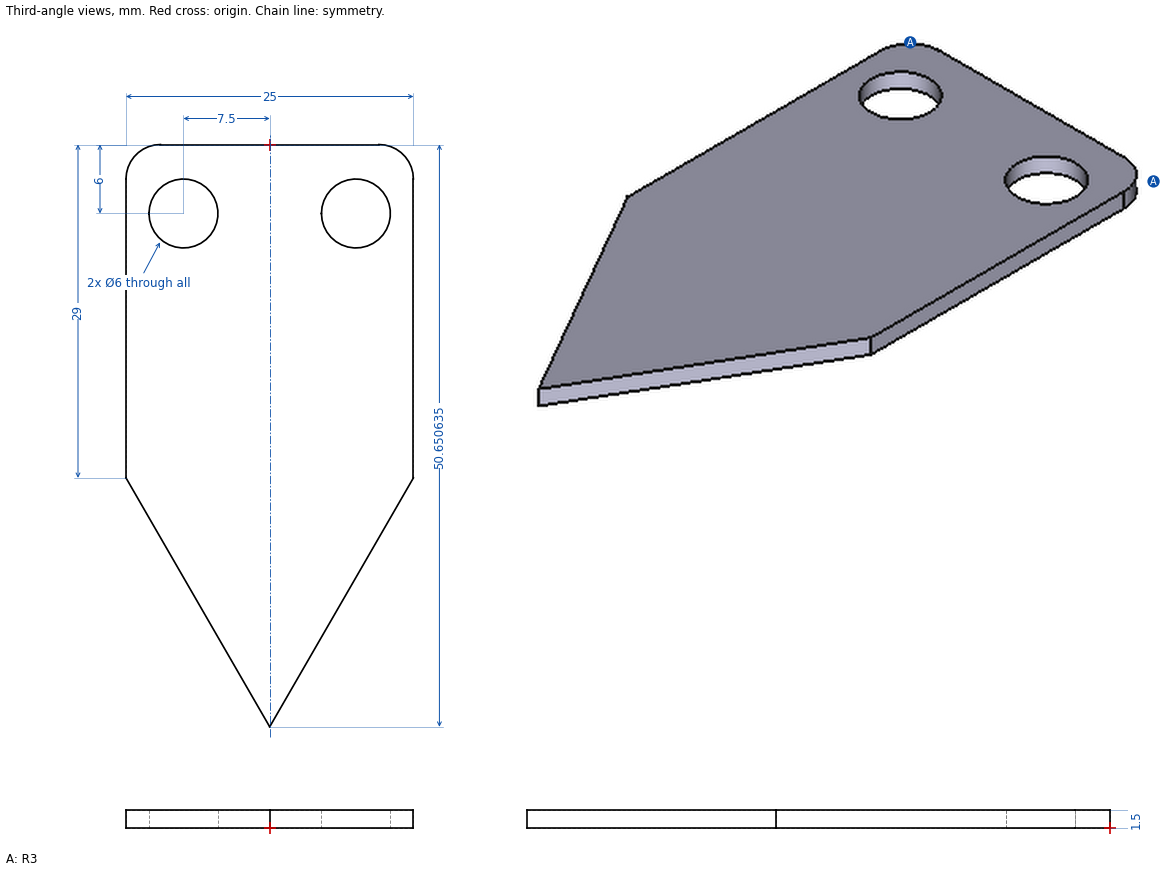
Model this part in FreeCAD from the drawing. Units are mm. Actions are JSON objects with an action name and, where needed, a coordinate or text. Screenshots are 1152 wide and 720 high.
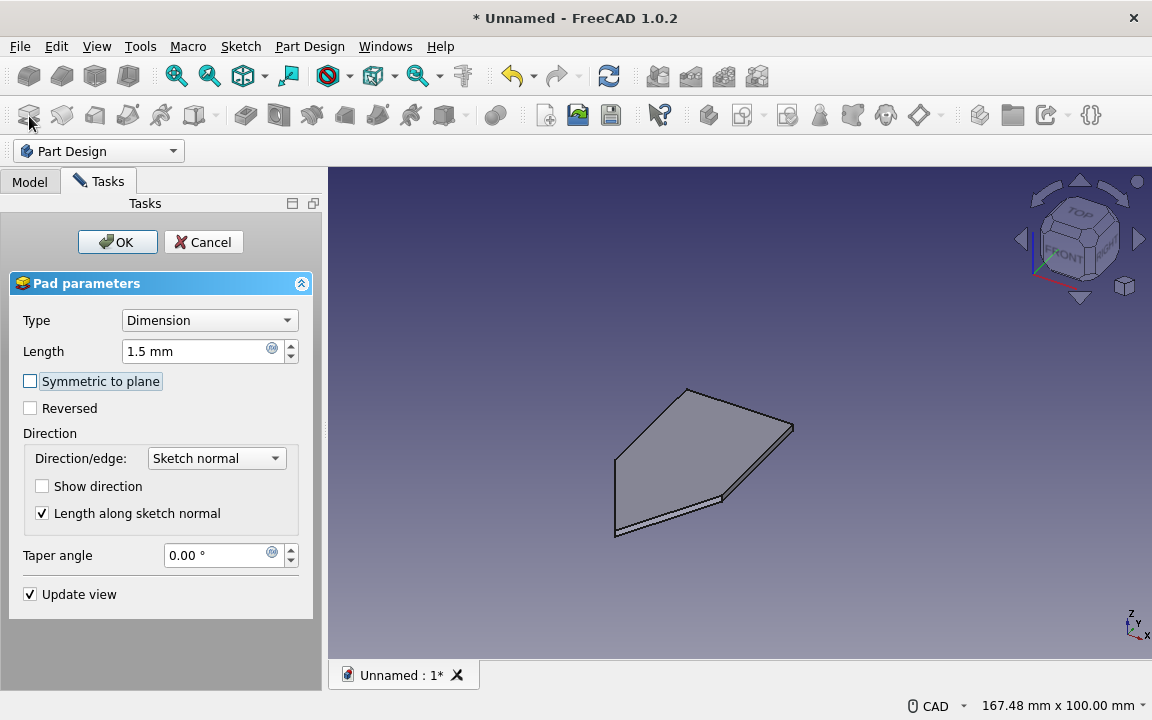
{"action": "left_click", "coordinate": [118, 242]}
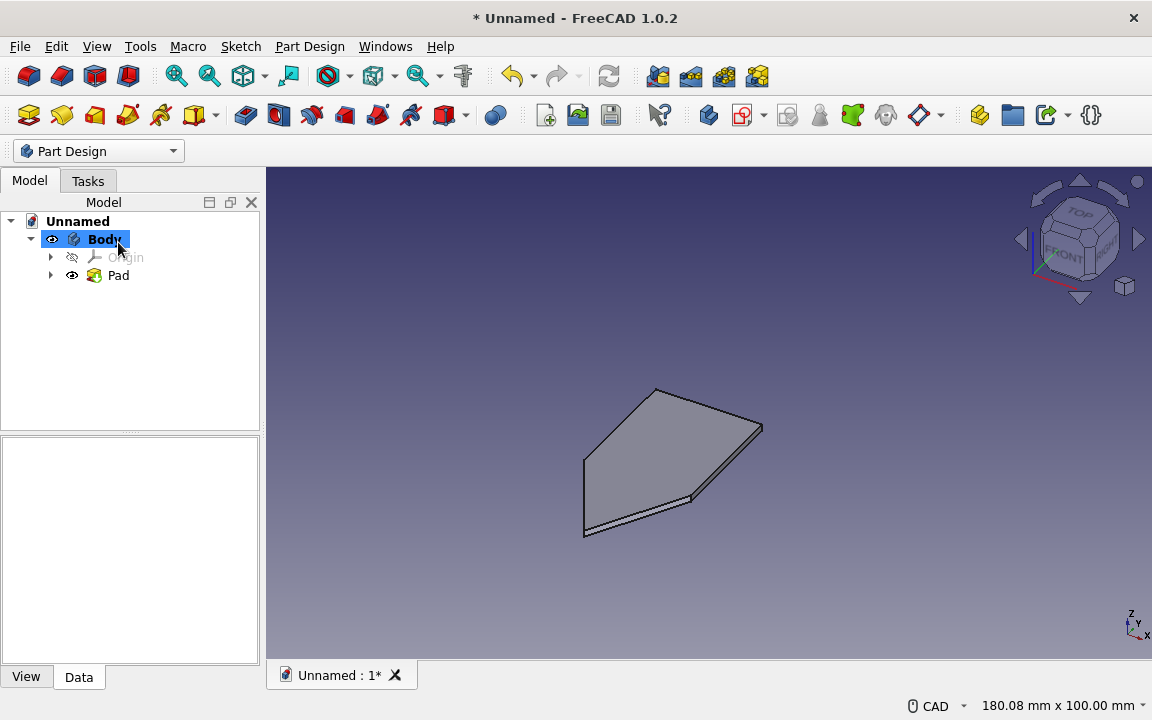
{"action": "left_click", "coordinate": [177, 76]}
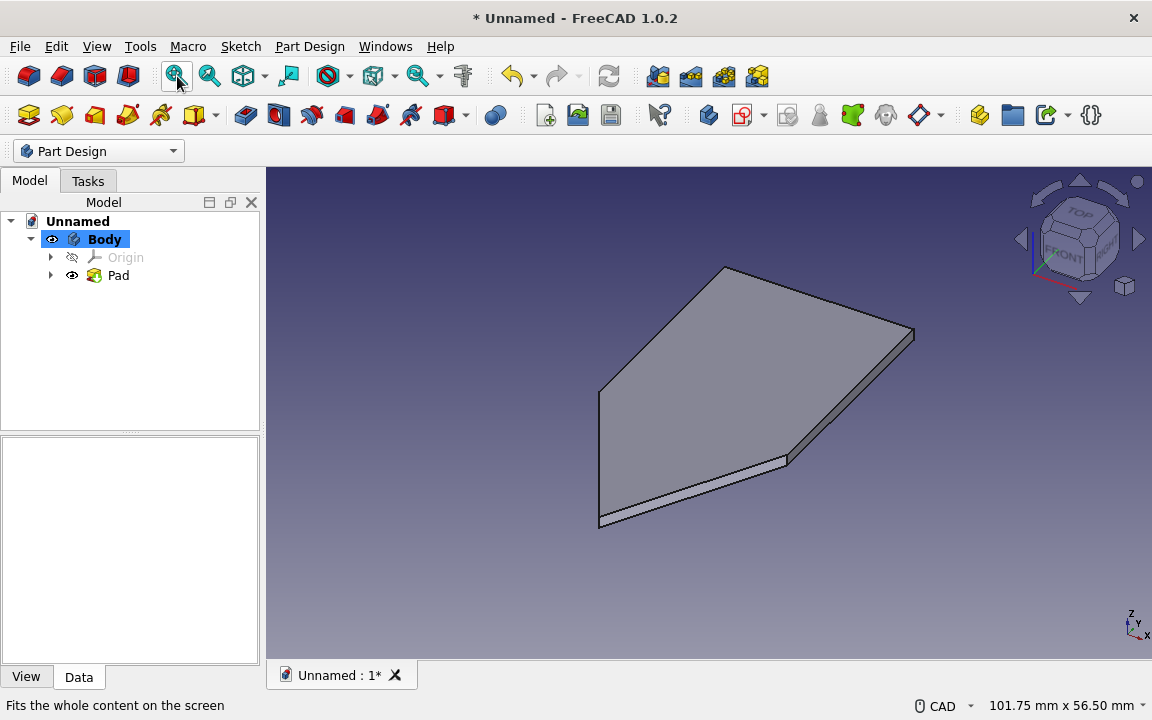
{"action": "left_click", "coordinate": [741, 375]}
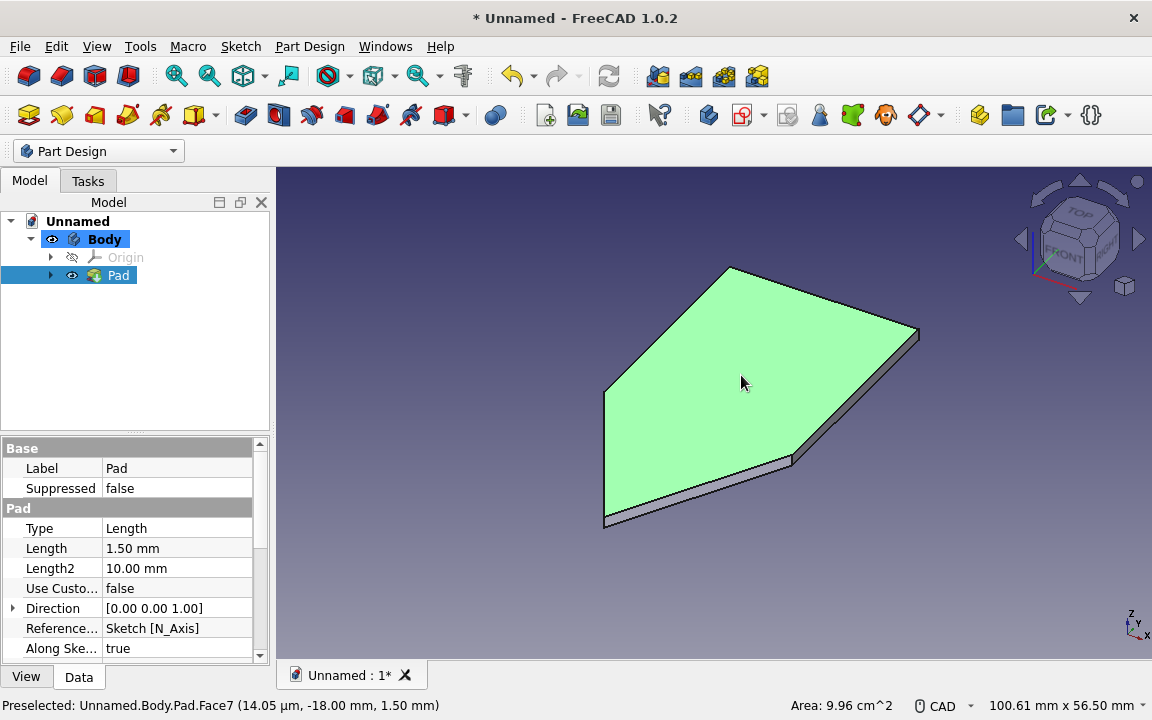
{"action": "left_click", "coordinate": [742, 116]}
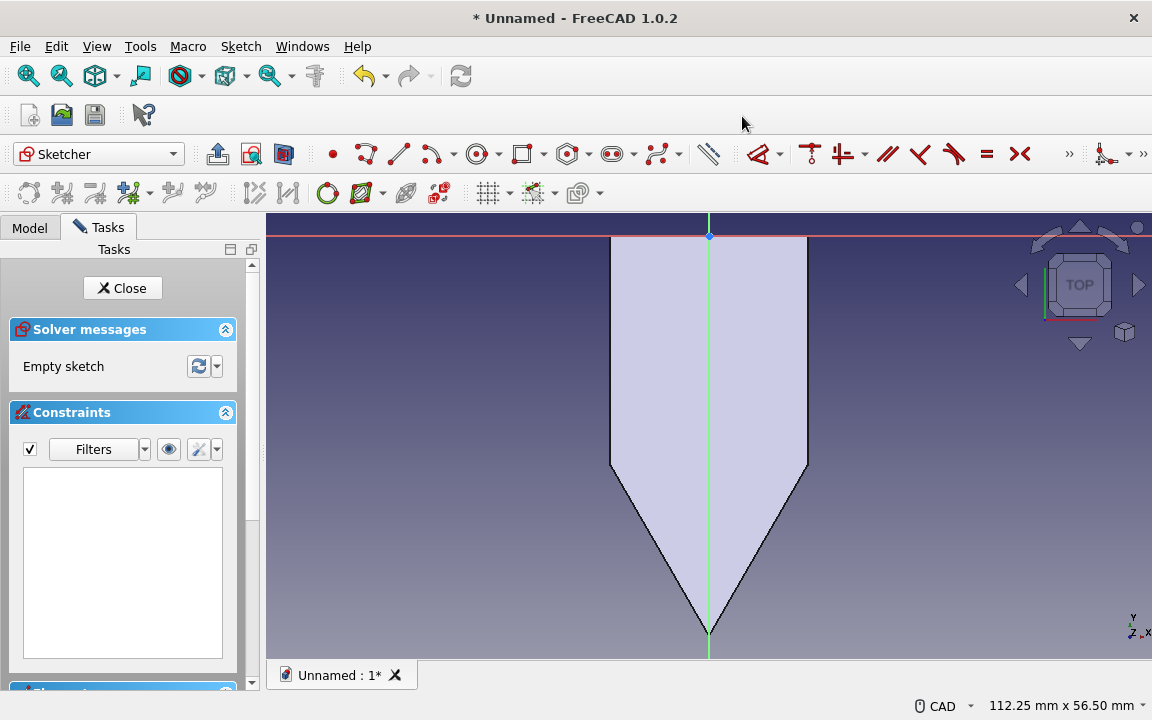
{"action": "scroll", "coordinate": [640, 436], "scroll_direction": "down", "scroll_amount": 5}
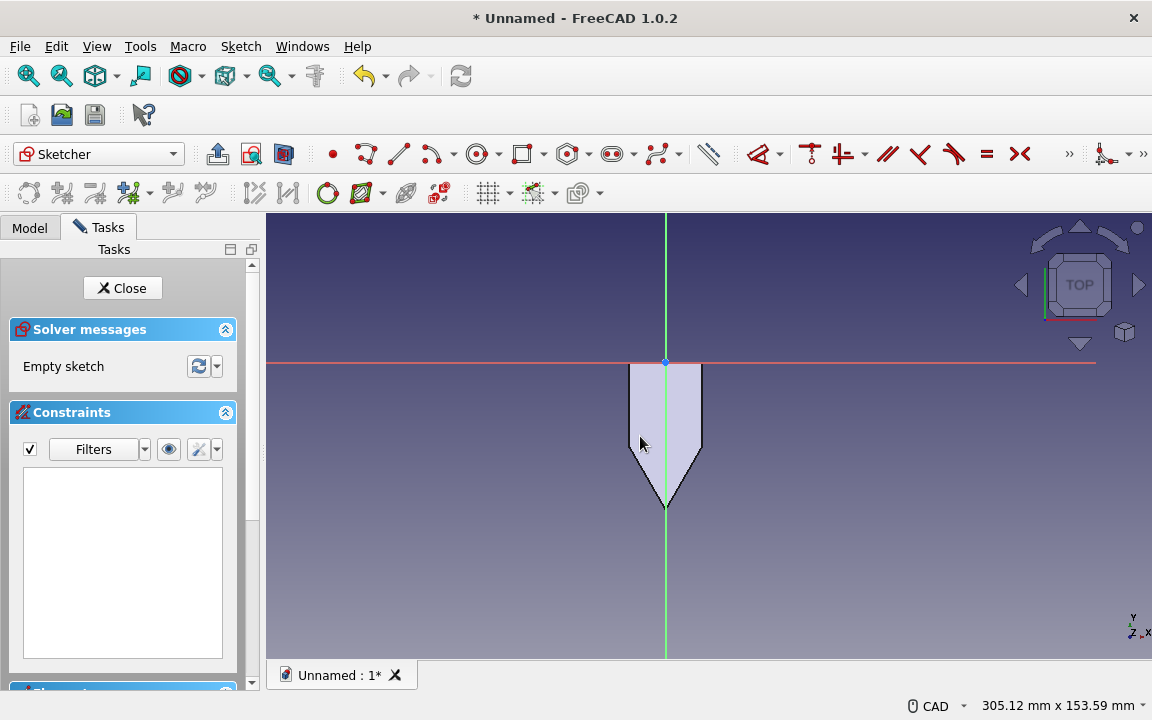
{"action": "scroll", "coordinate": [670, 366], "scroll_direction": "up", "scroll_amount": 10}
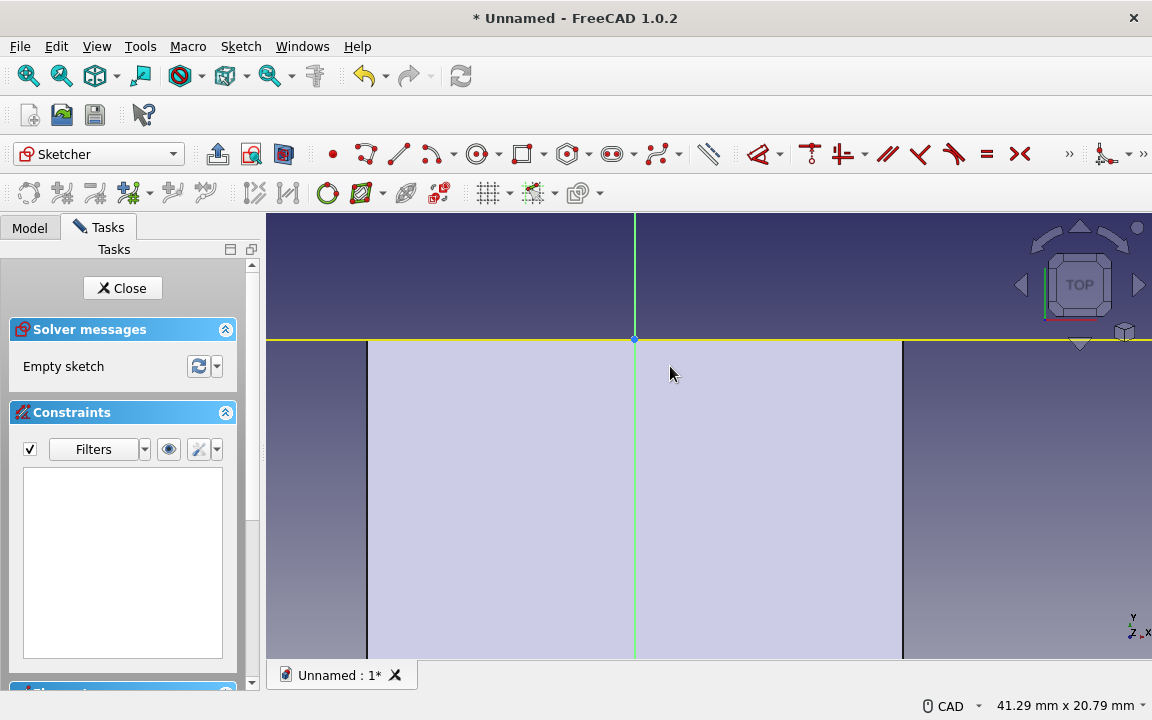
{"action": "left_click", "coordinate": [476, 154]}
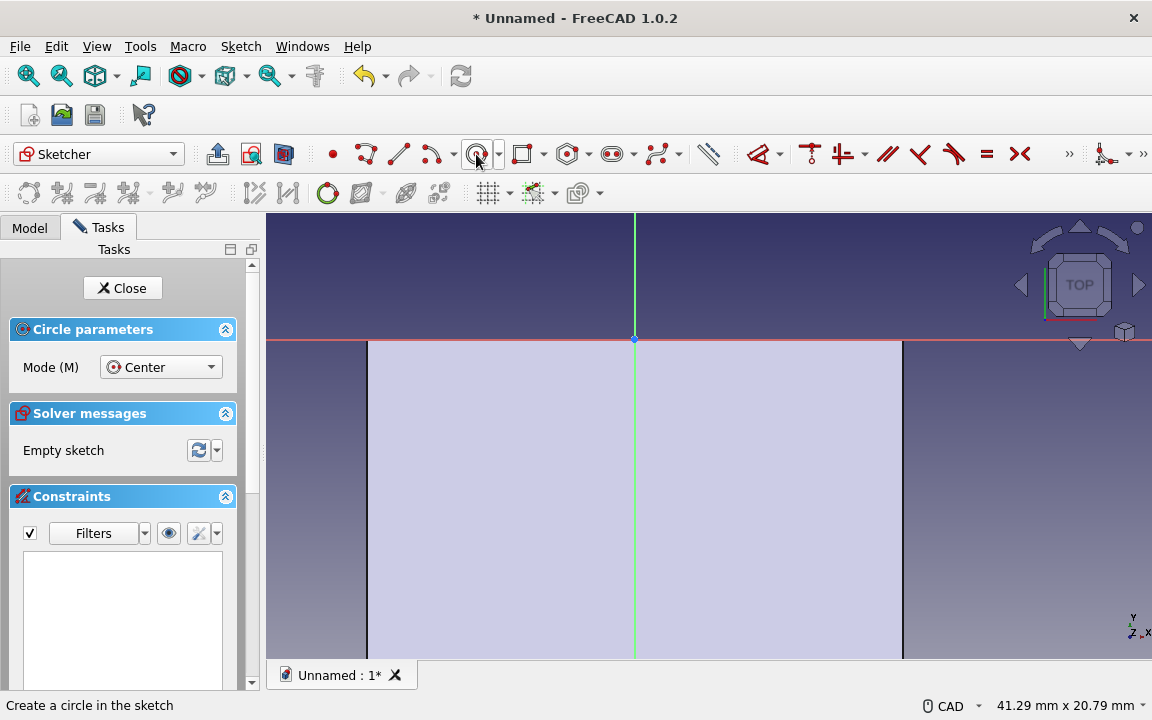
{"action": "left_click", "coordinate": [474, 469]}
{"action": "left_click", "coordinate": [520, 423]}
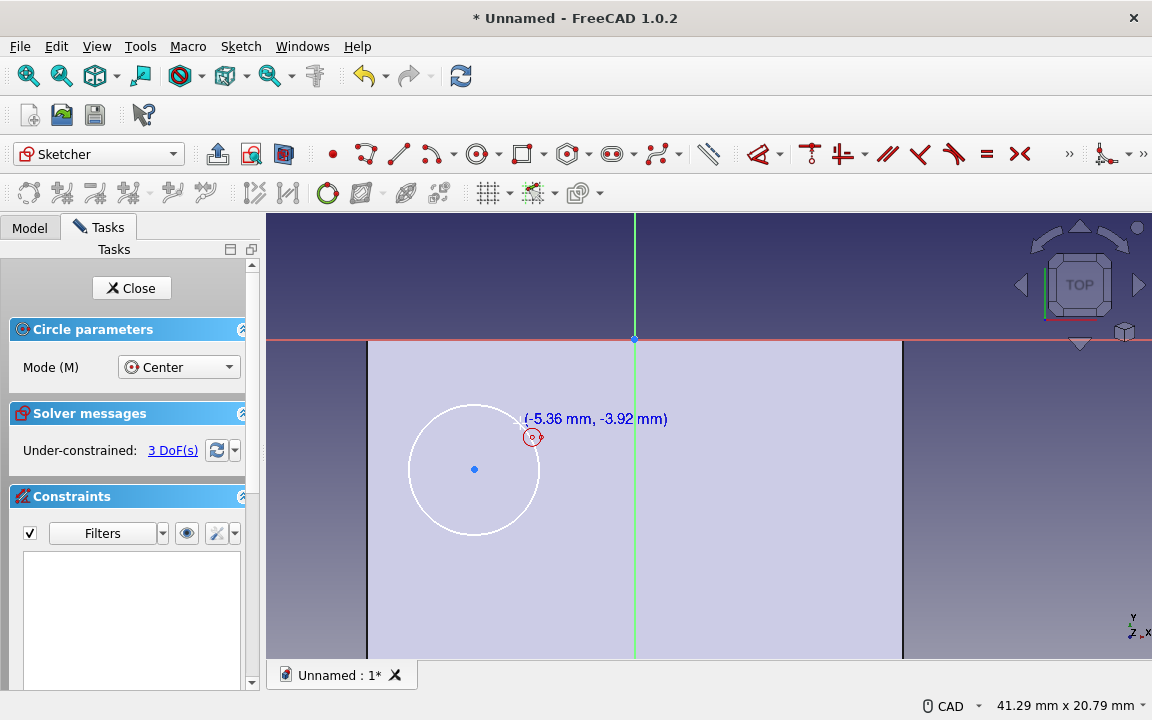
{"action": "left_click", "coordinate": [796, 469]}
{"action": "left_click", "coordinate": [841, 423]}
{"action": "key", "text": "Escape"}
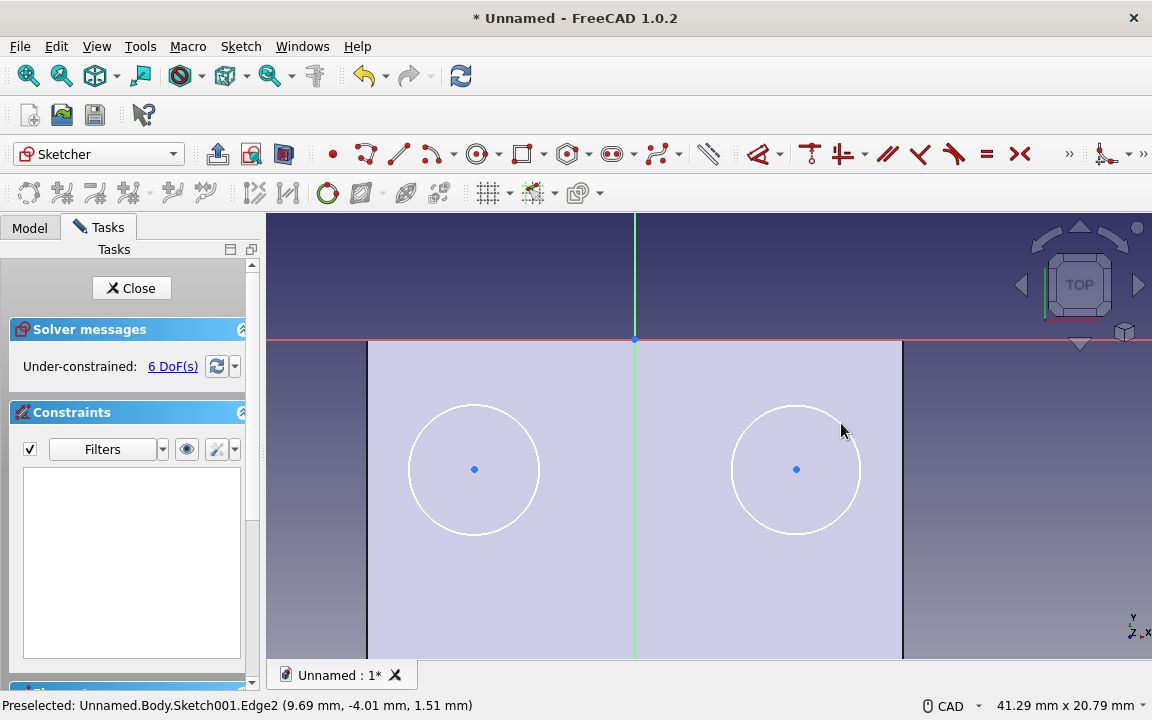
{"action": "left_click", "coordinate": [520, 424]}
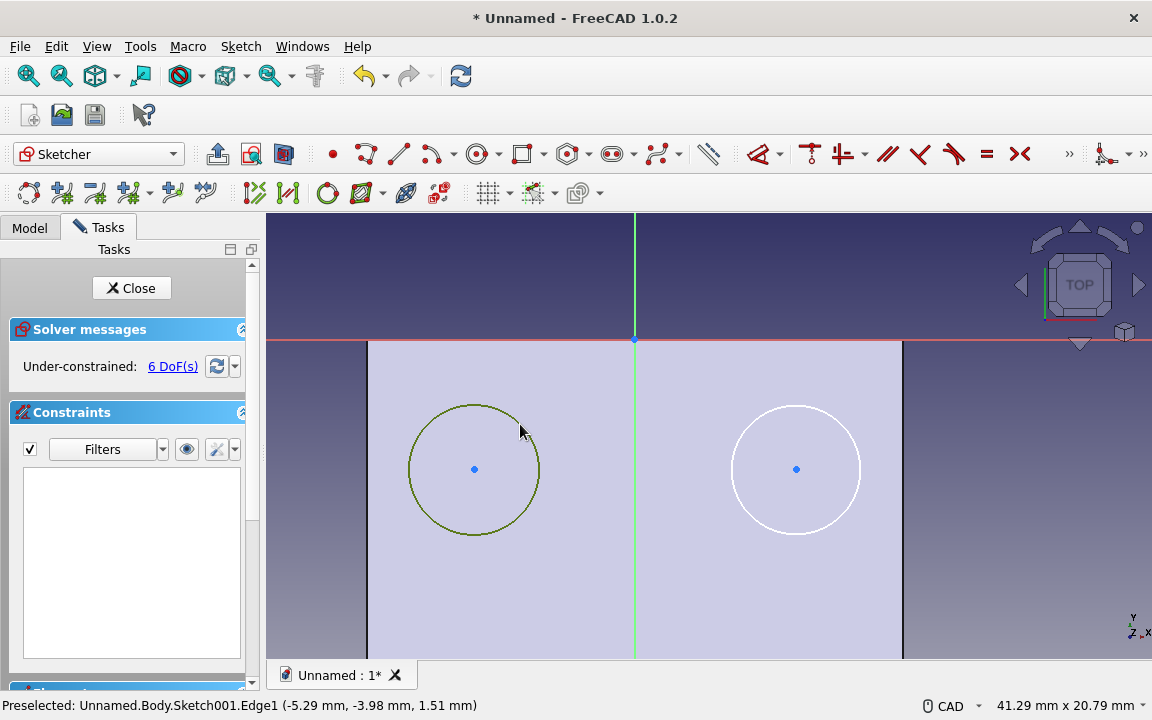
{"action": "left_click", "coordinate": [841, 424]}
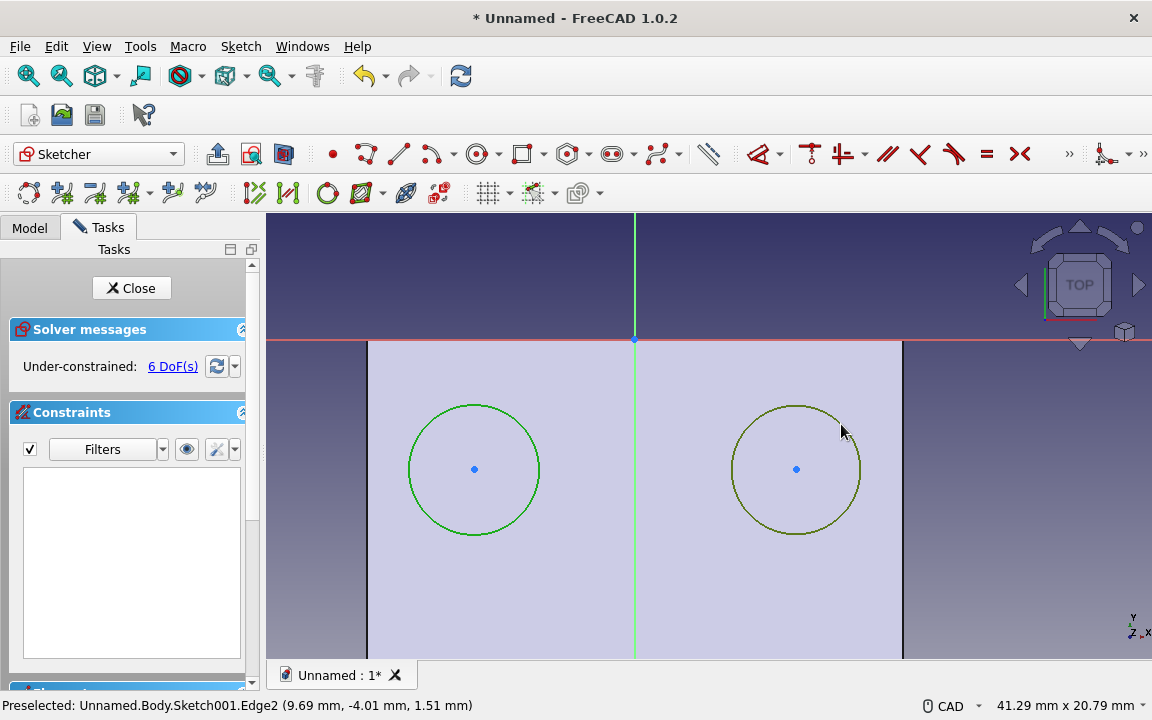
{"action": "left_click", "coordinate": [987, 154]}